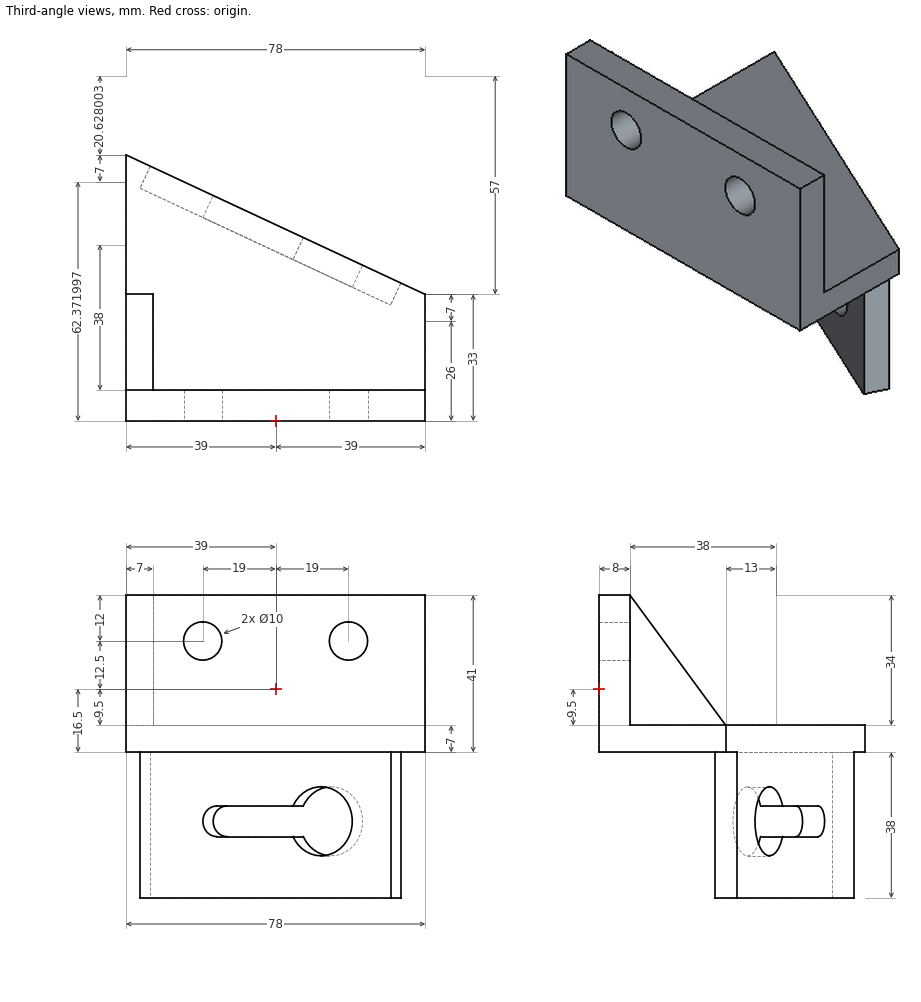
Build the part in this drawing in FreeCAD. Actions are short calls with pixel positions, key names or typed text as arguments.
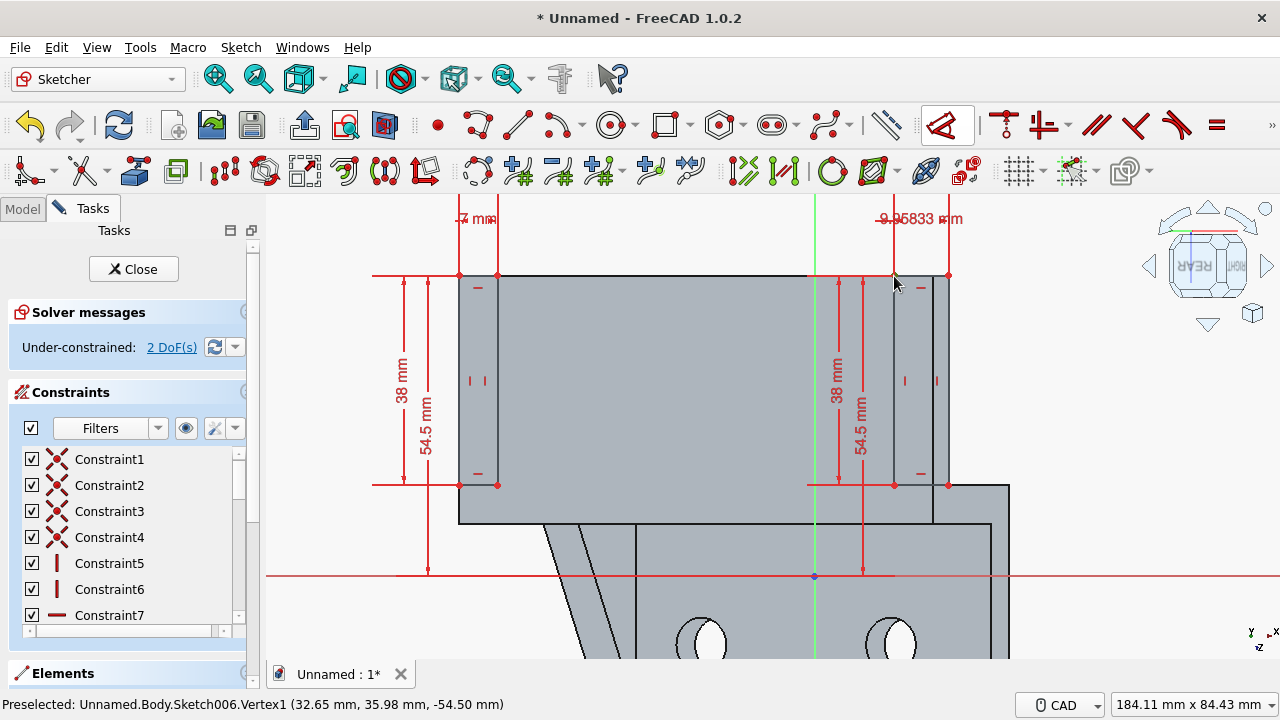
key(l)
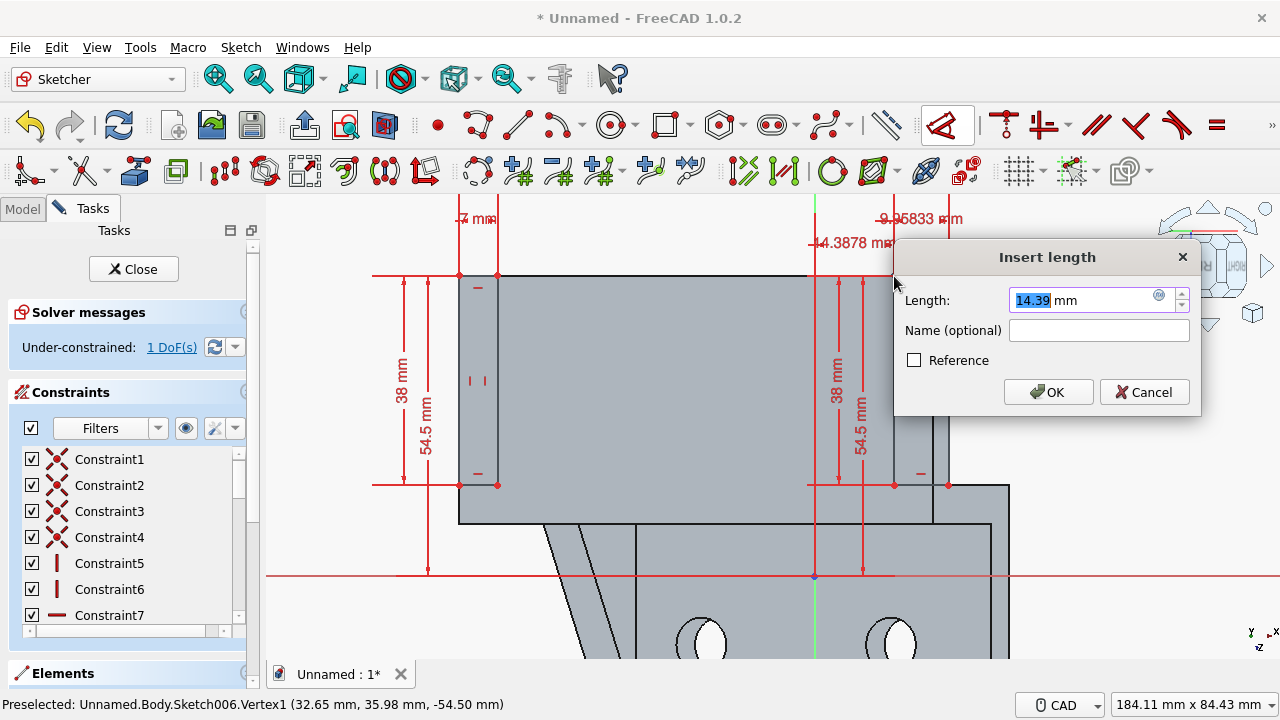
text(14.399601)
key(Return)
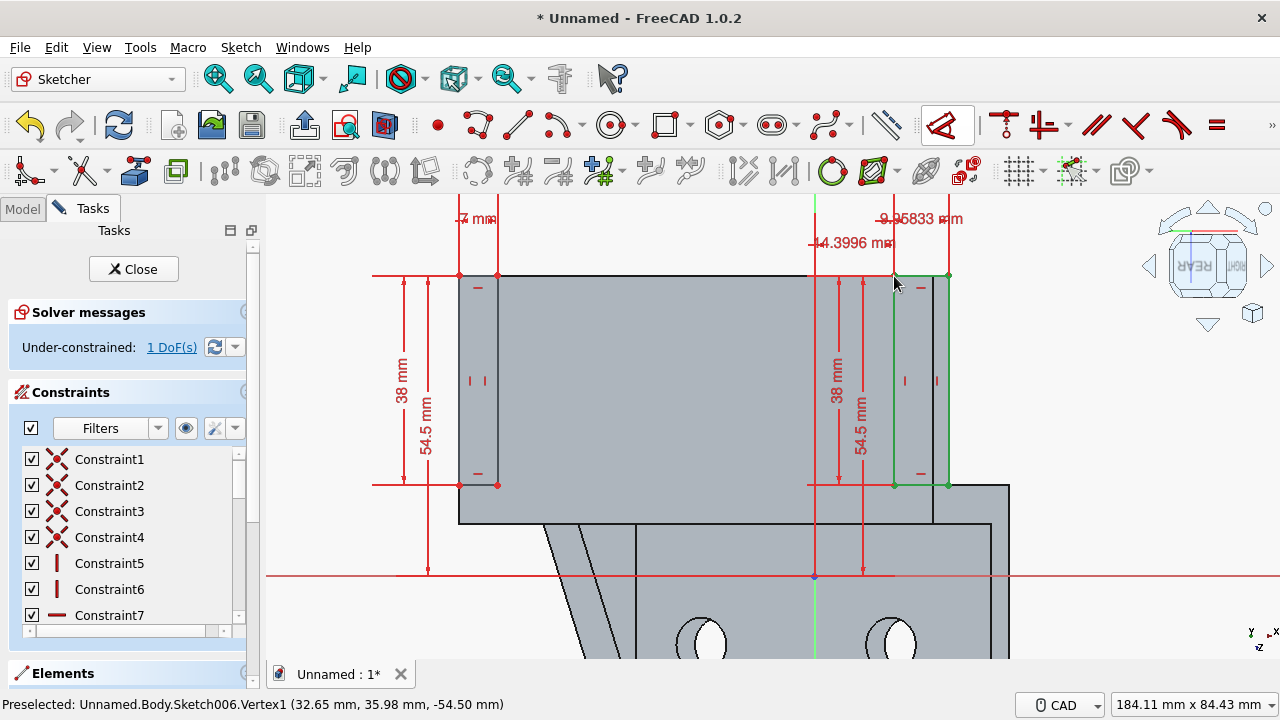
click(459, 276)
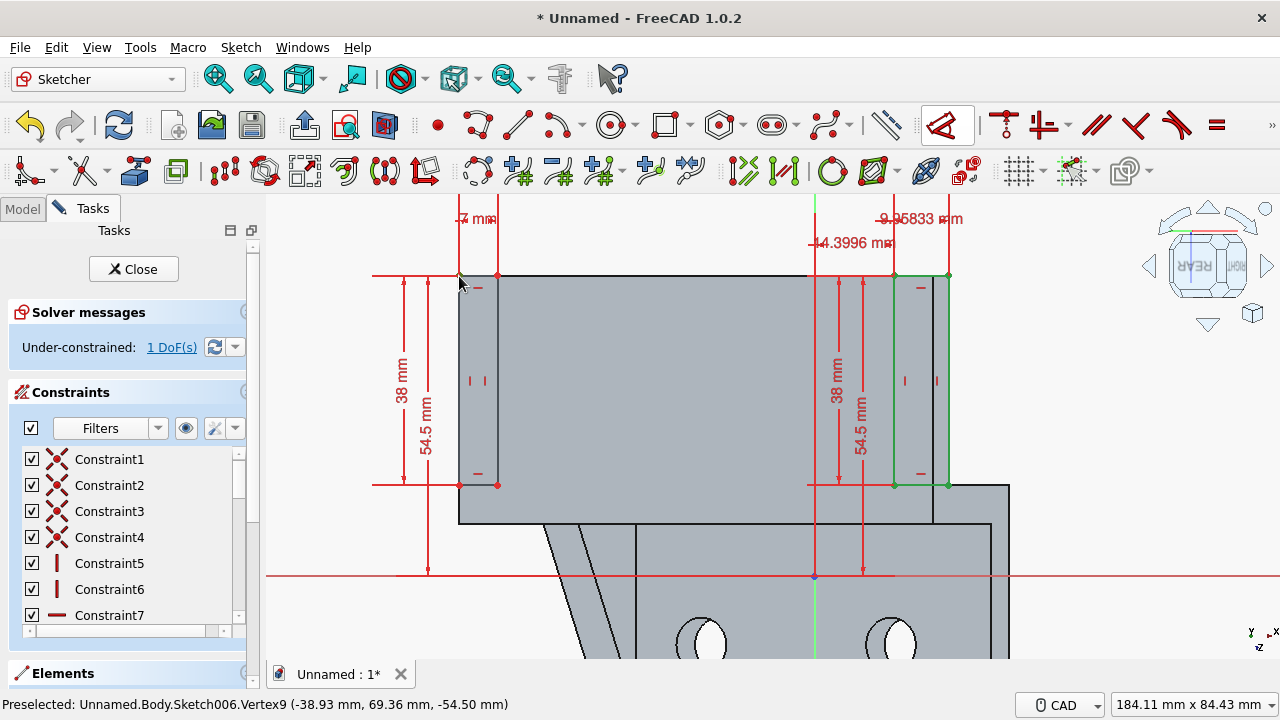
key(l)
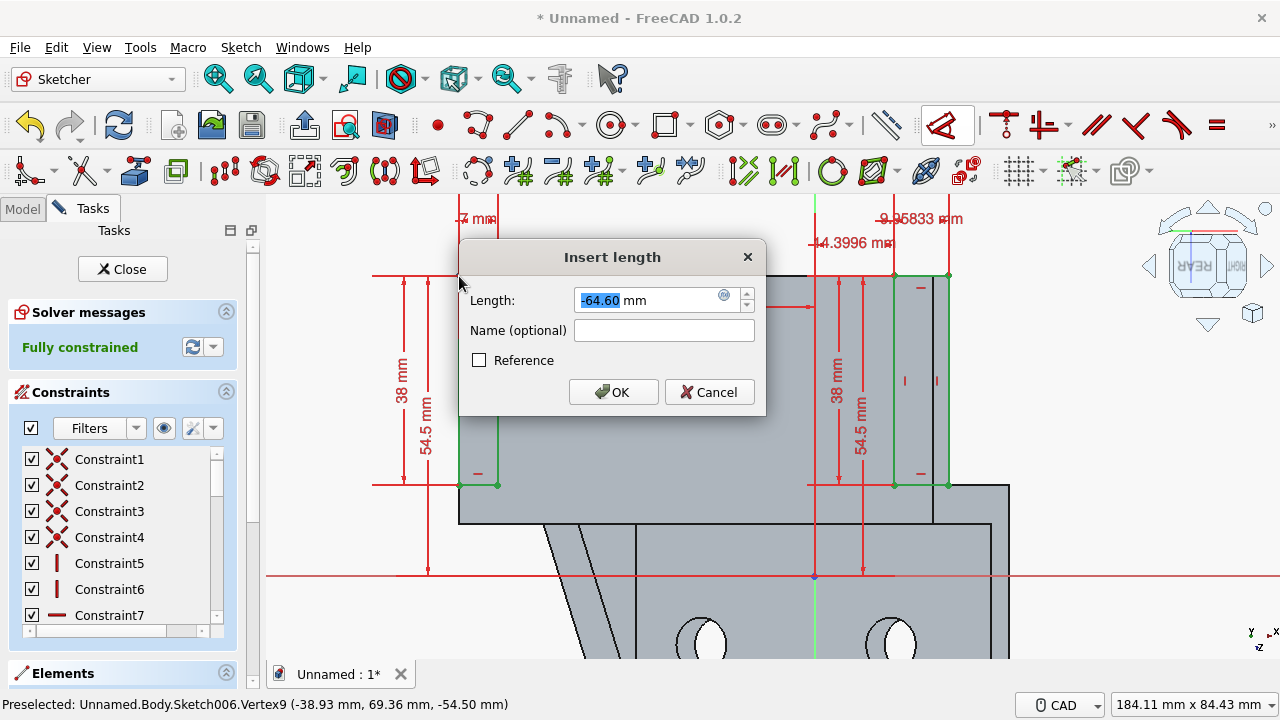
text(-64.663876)
key(Return)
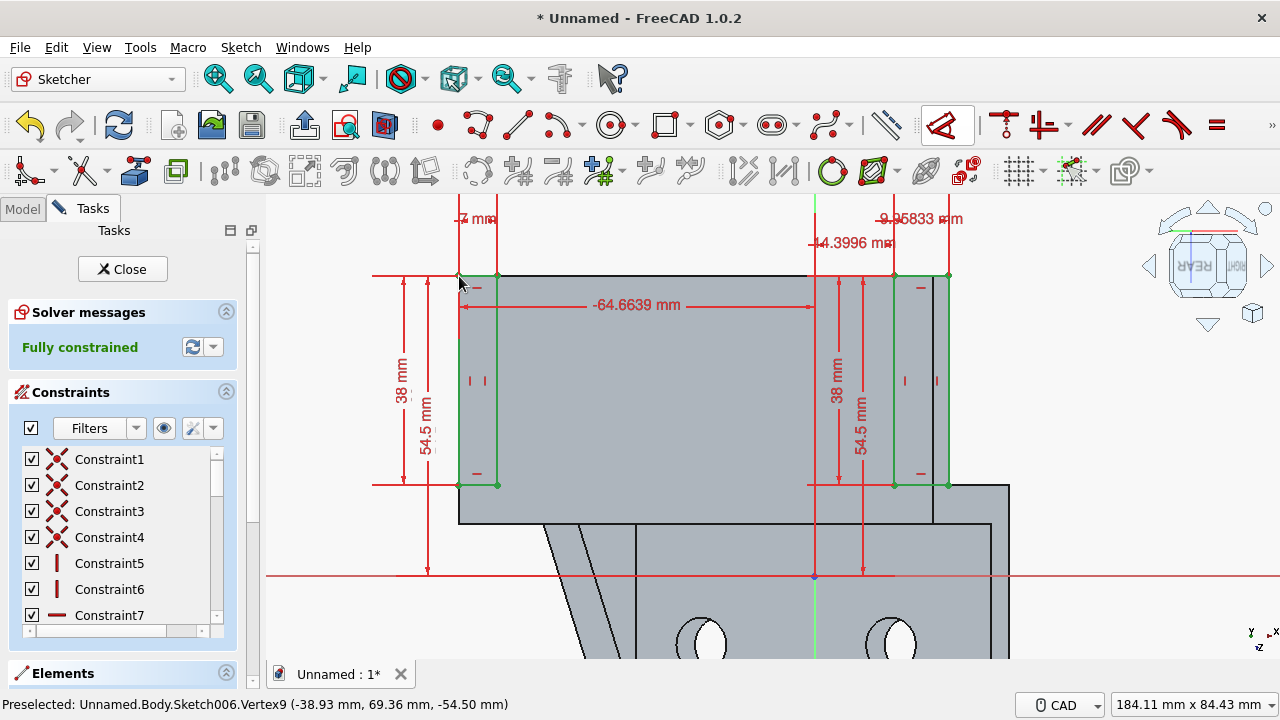
click(123, 269)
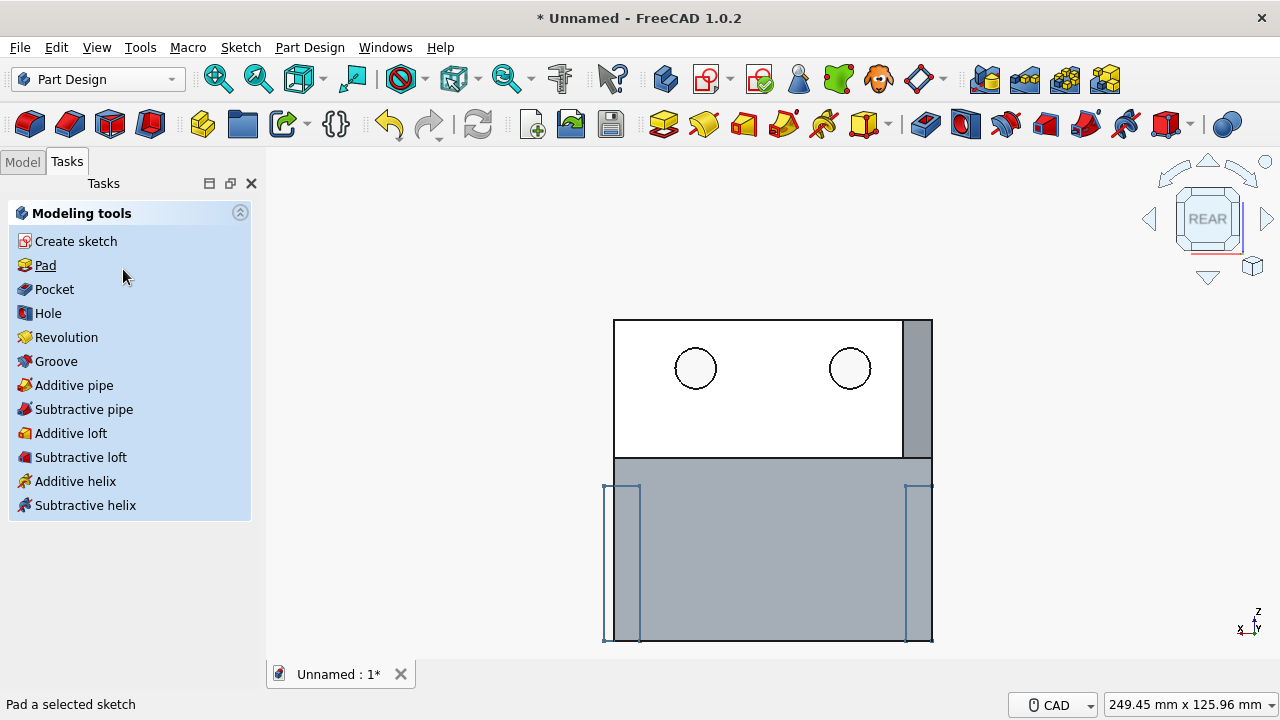
click(926, 124)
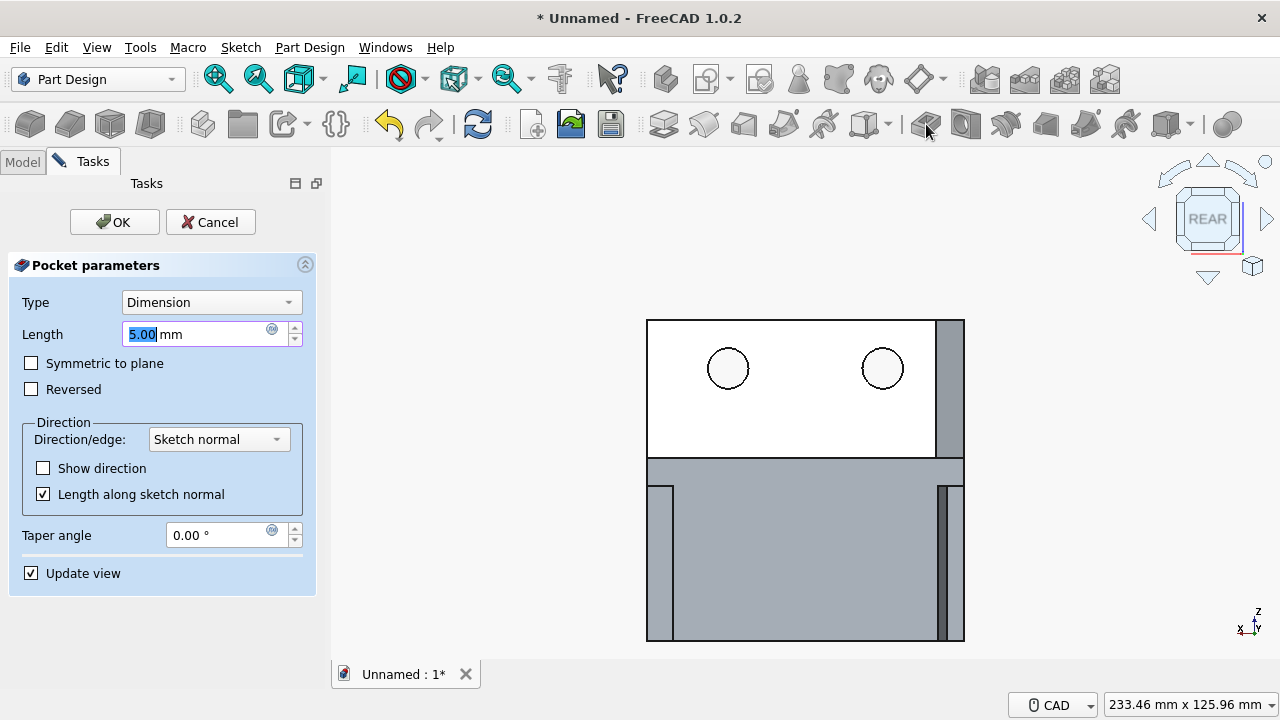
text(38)
key(Tab)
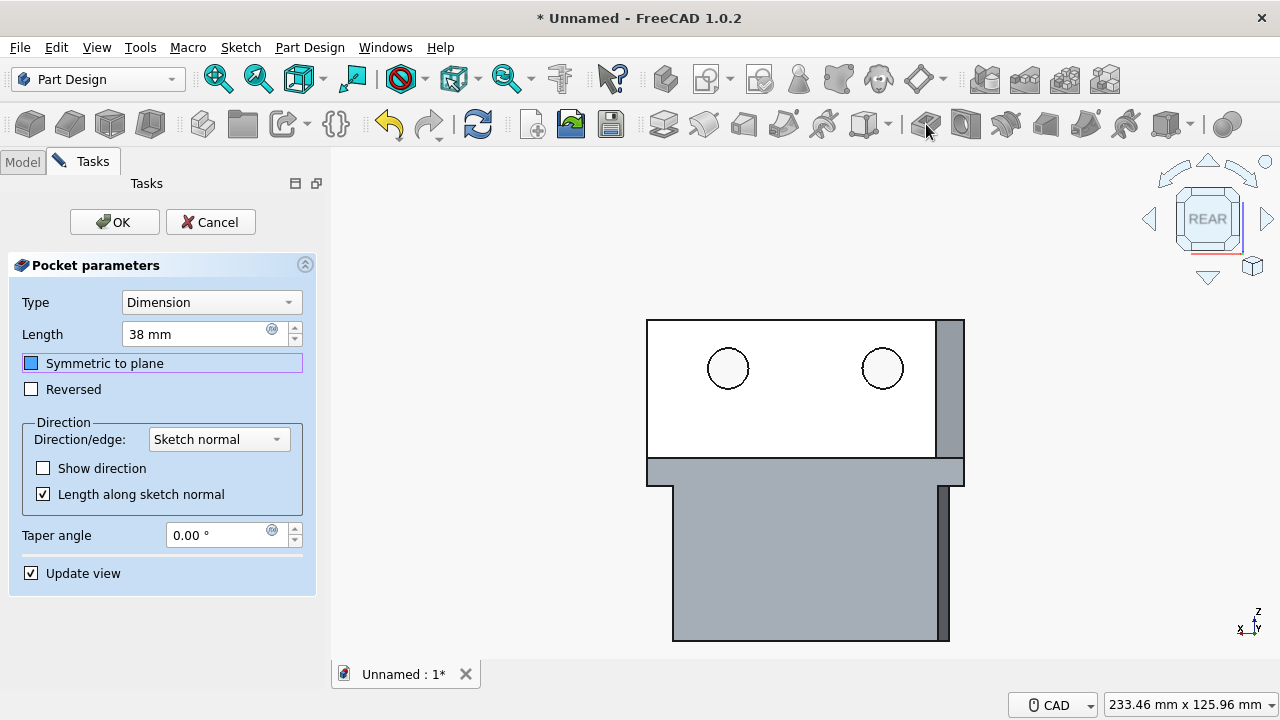
click(115, 222)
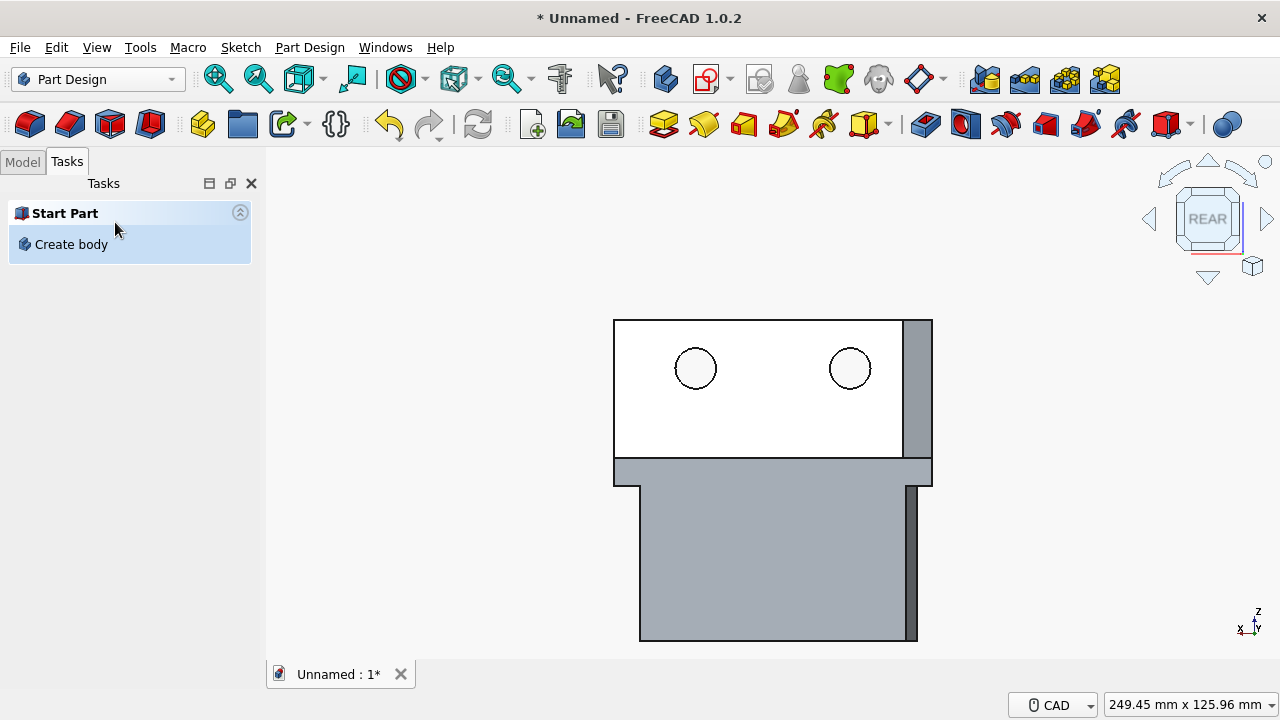
click(728, 548)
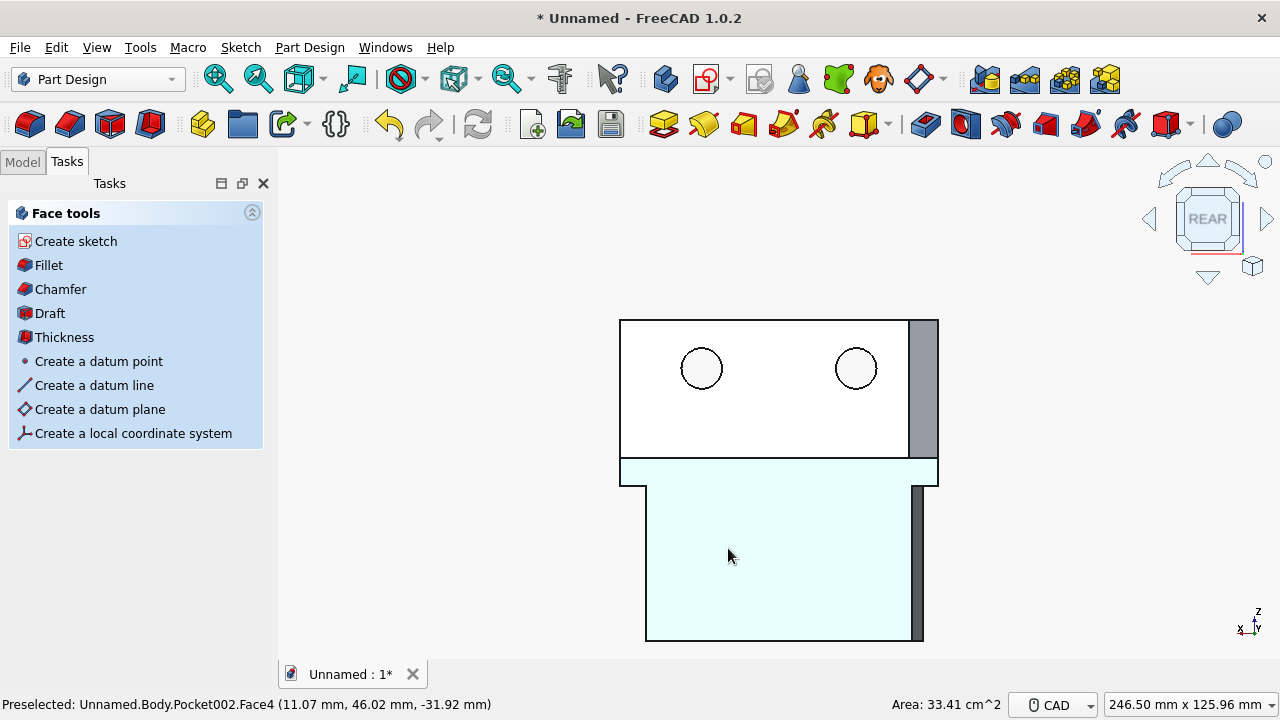
click(706, 80)